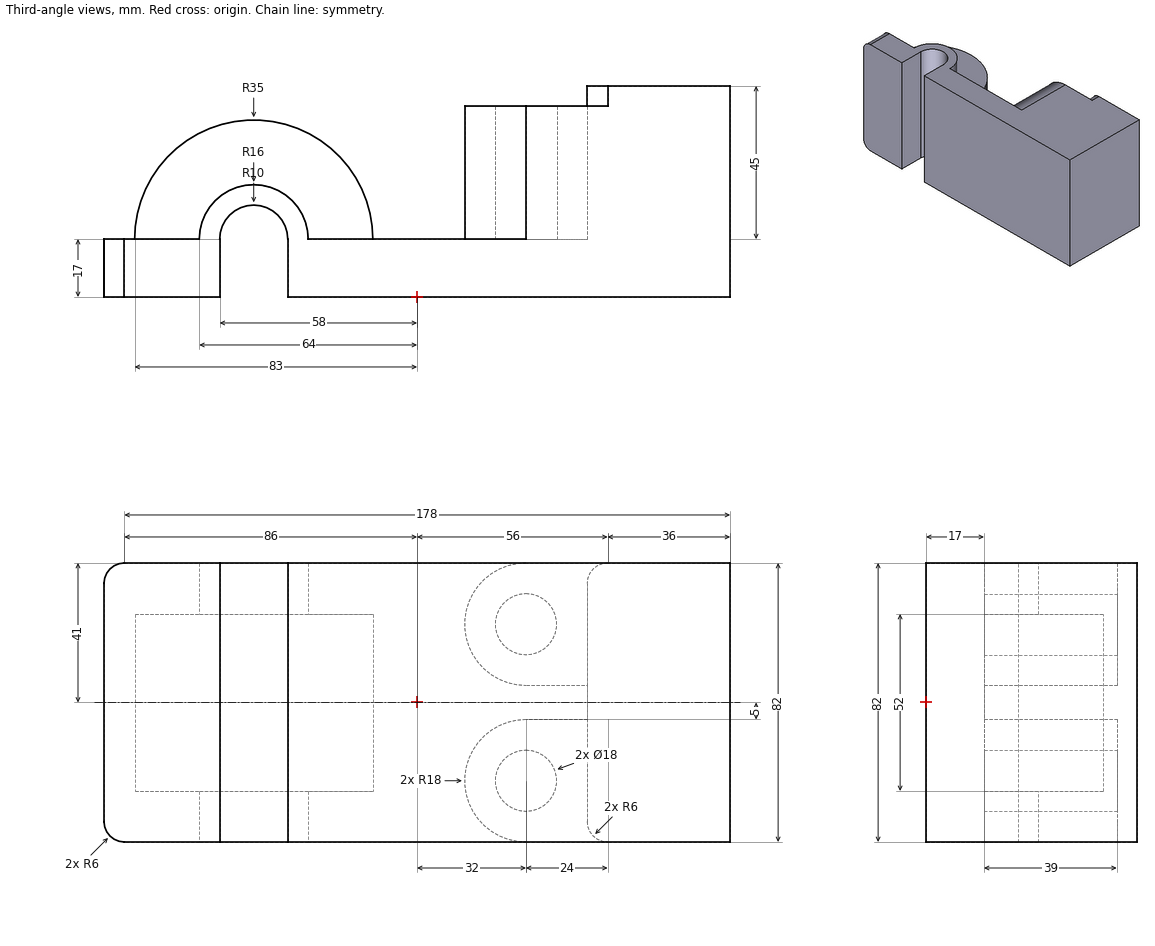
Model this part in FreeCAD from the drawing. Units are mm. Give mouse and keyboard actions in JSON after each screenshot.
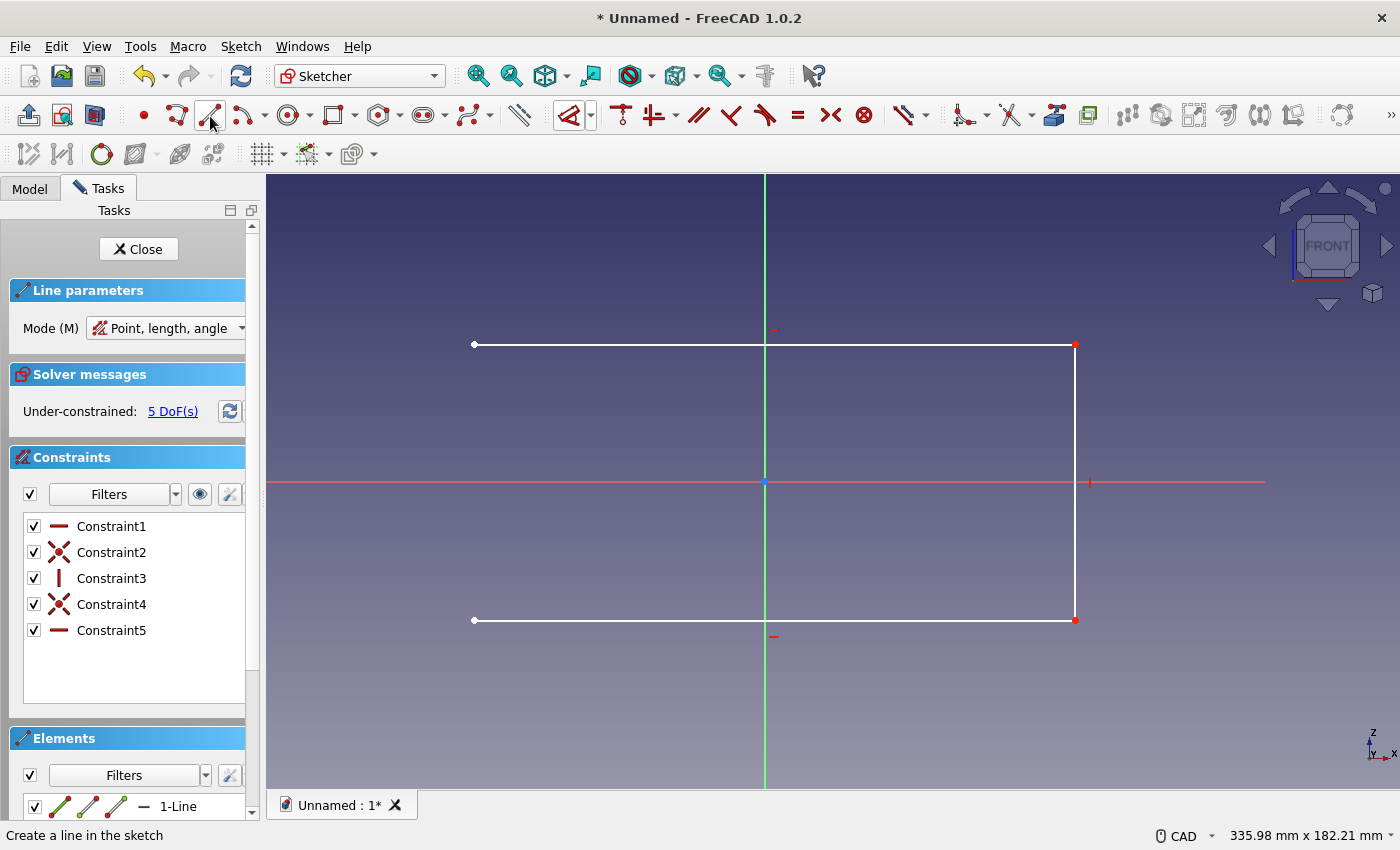
{"action": "left_click", "coordinate": [454, 600]}
{"action": "left_click", "coordinate": [454, 364]}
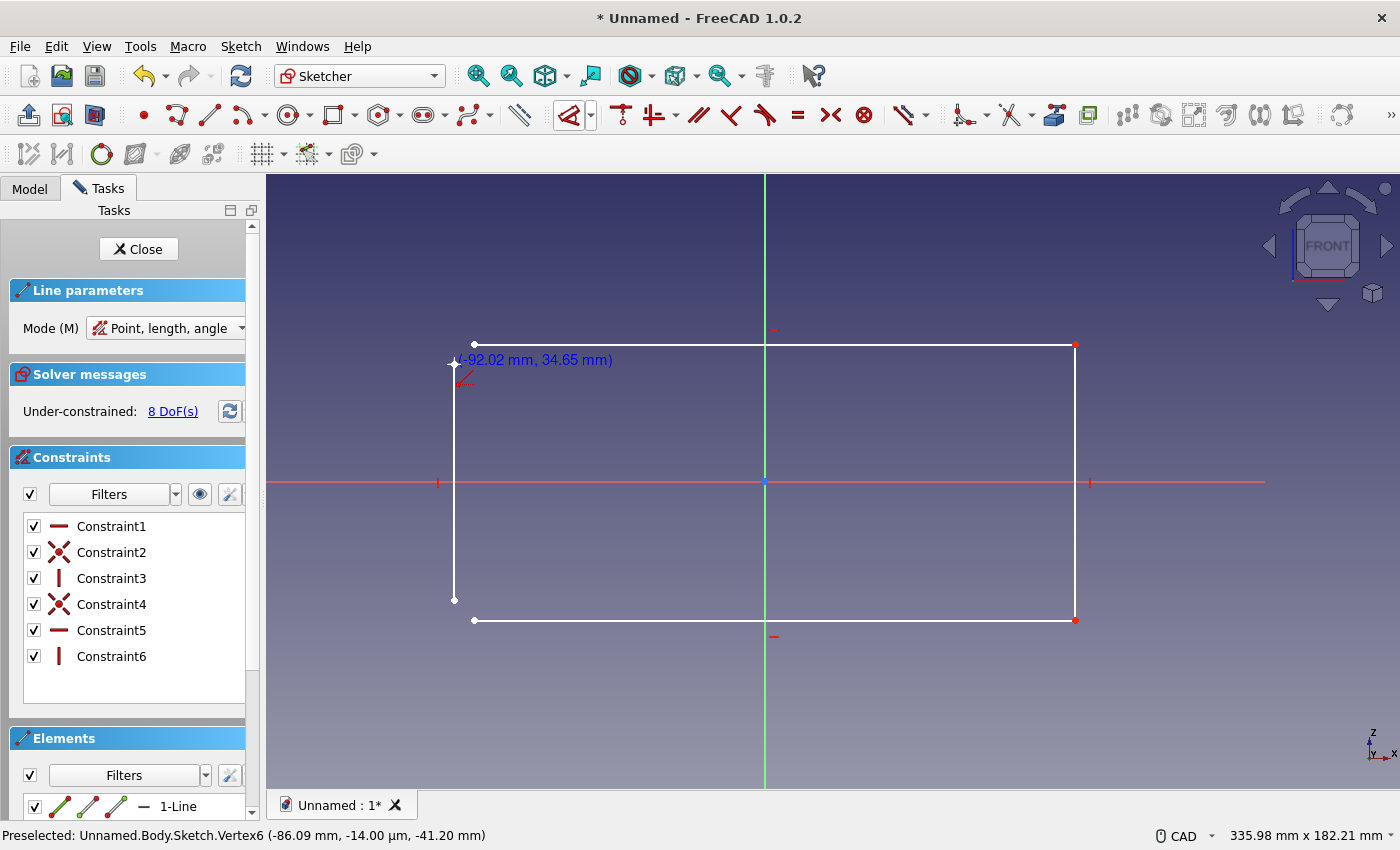
{"action": "key", "text": "g 3 a"}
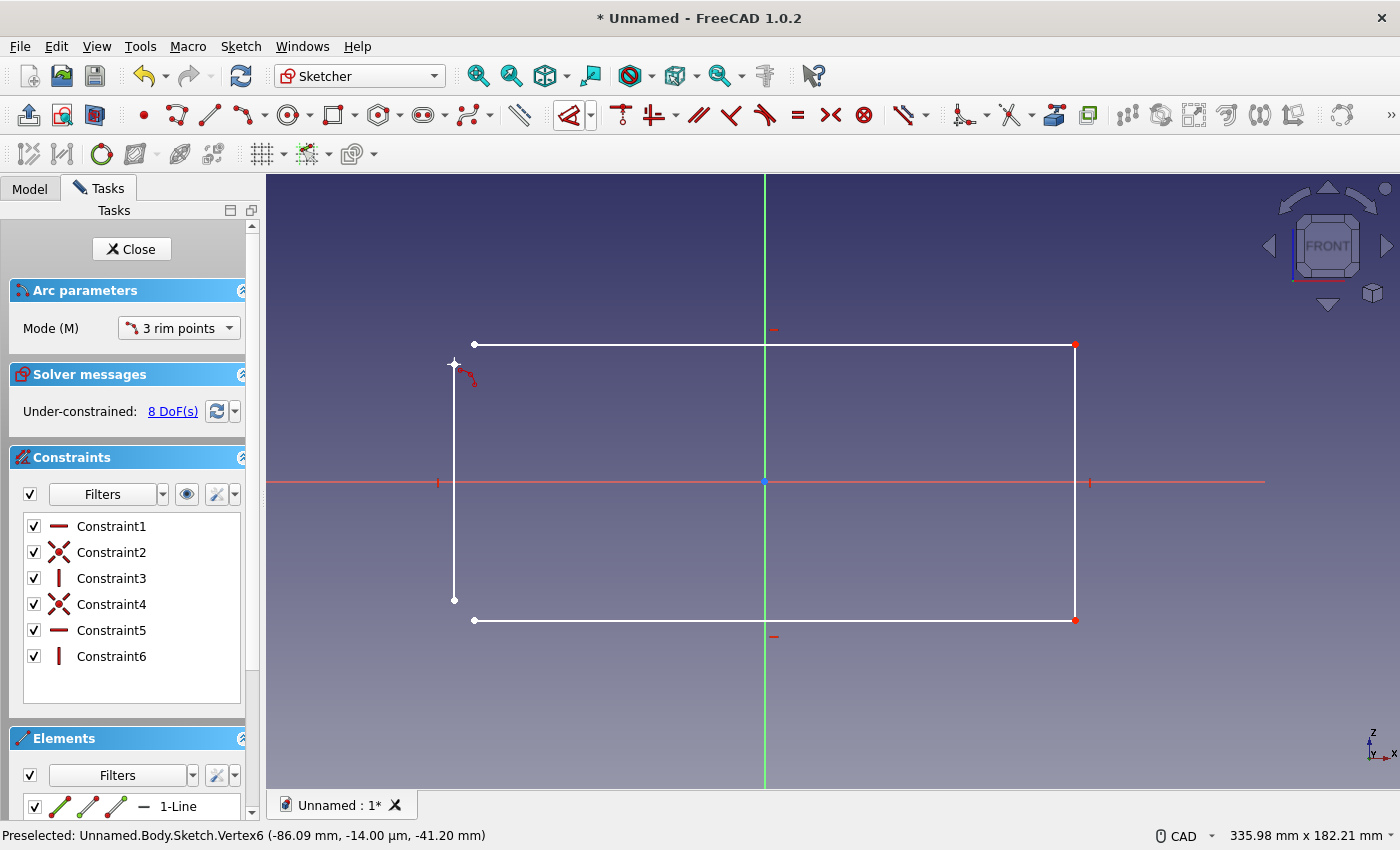
{"action": "left_click", "coordinate": [474, 621]}
{"action": "left_click", "coordinate": [454, 601]}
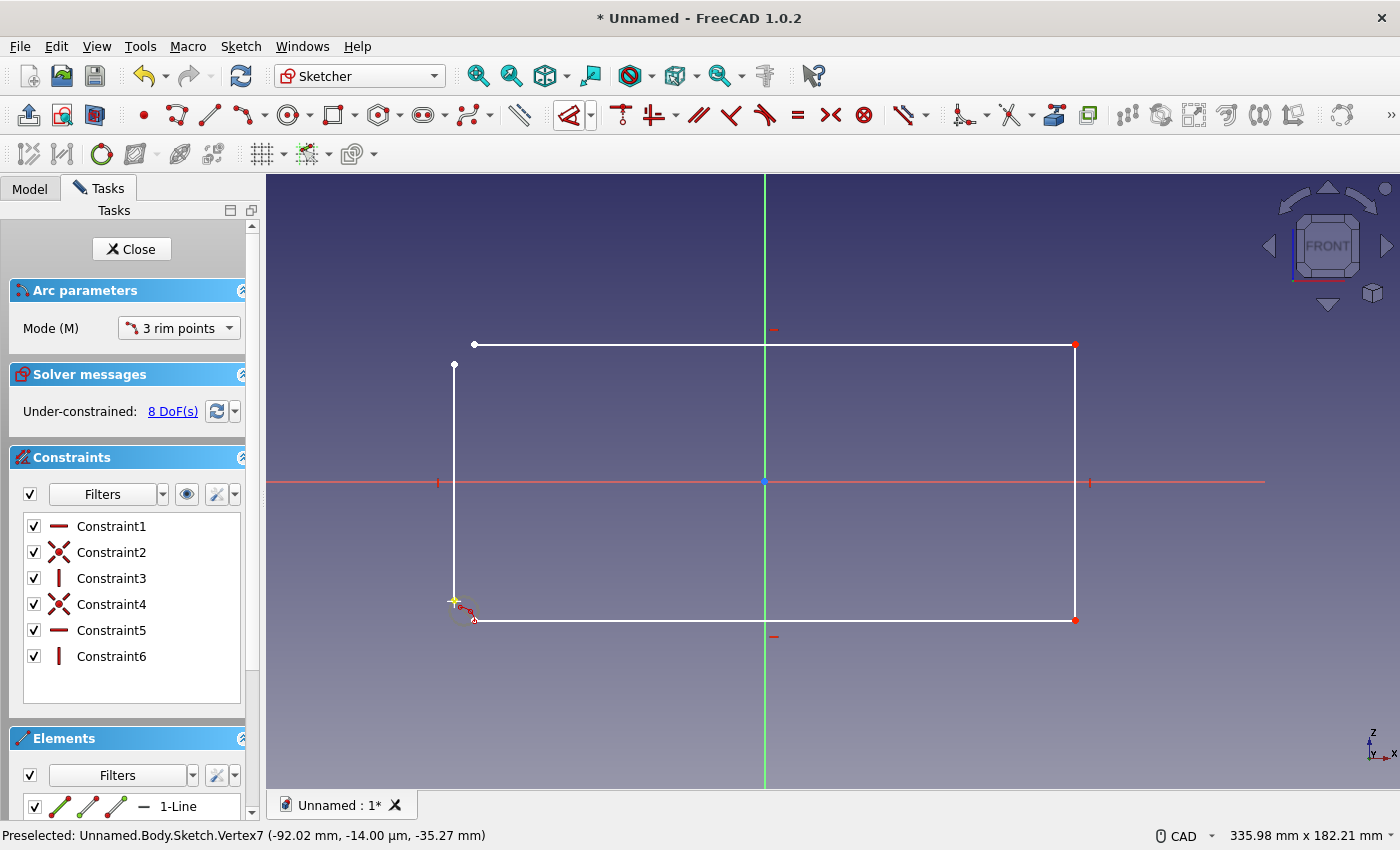
{"action": "scroll", "coordinate": [460, 614], "scroll_direction": "up", "scroll_amount": 5}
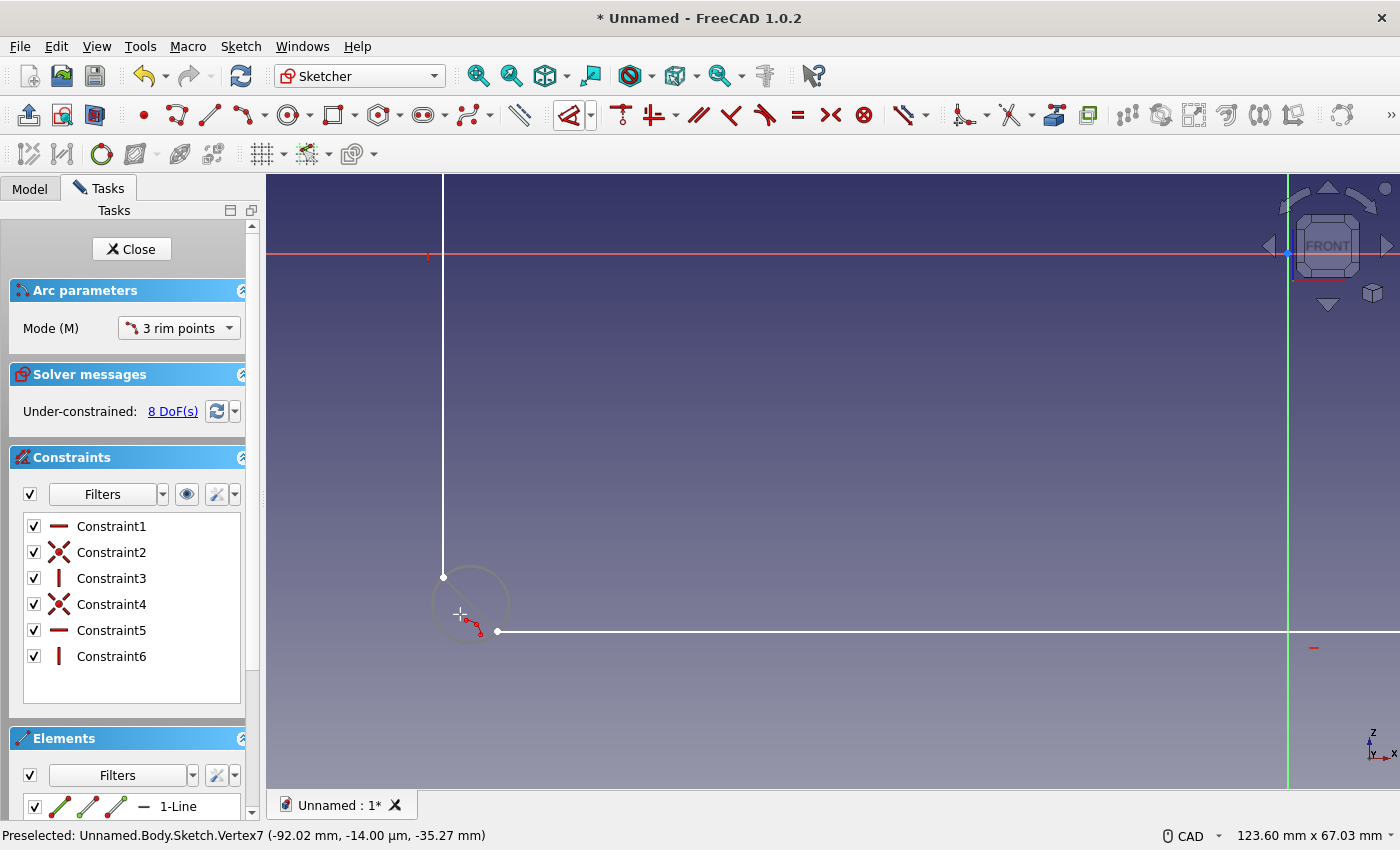
{"action": "left_click", "coordinate": [460, 614]}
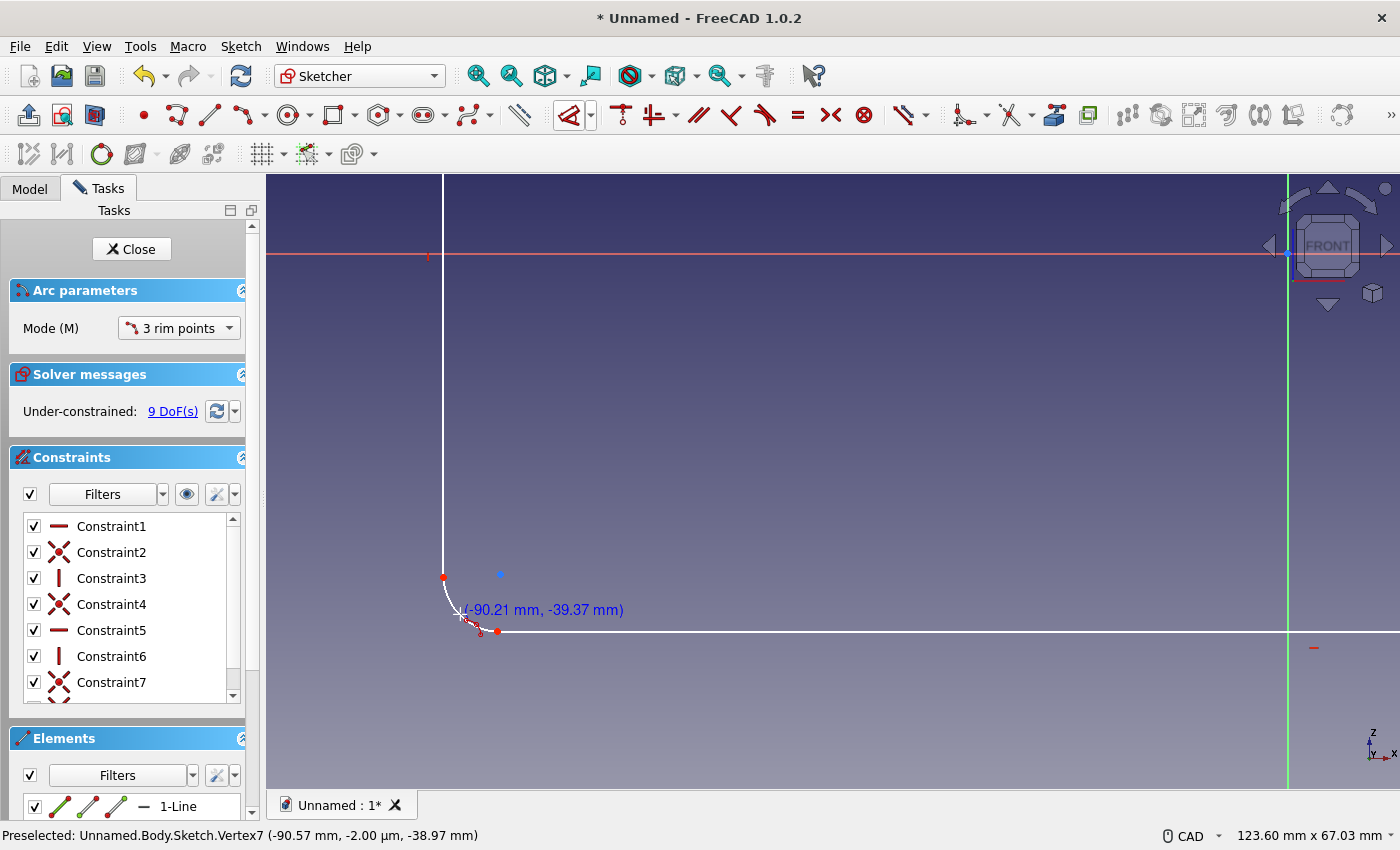
{"action": "scroll", "coordinate": [460, 614], "scroll_direction": "down", "scroll_amount": 5}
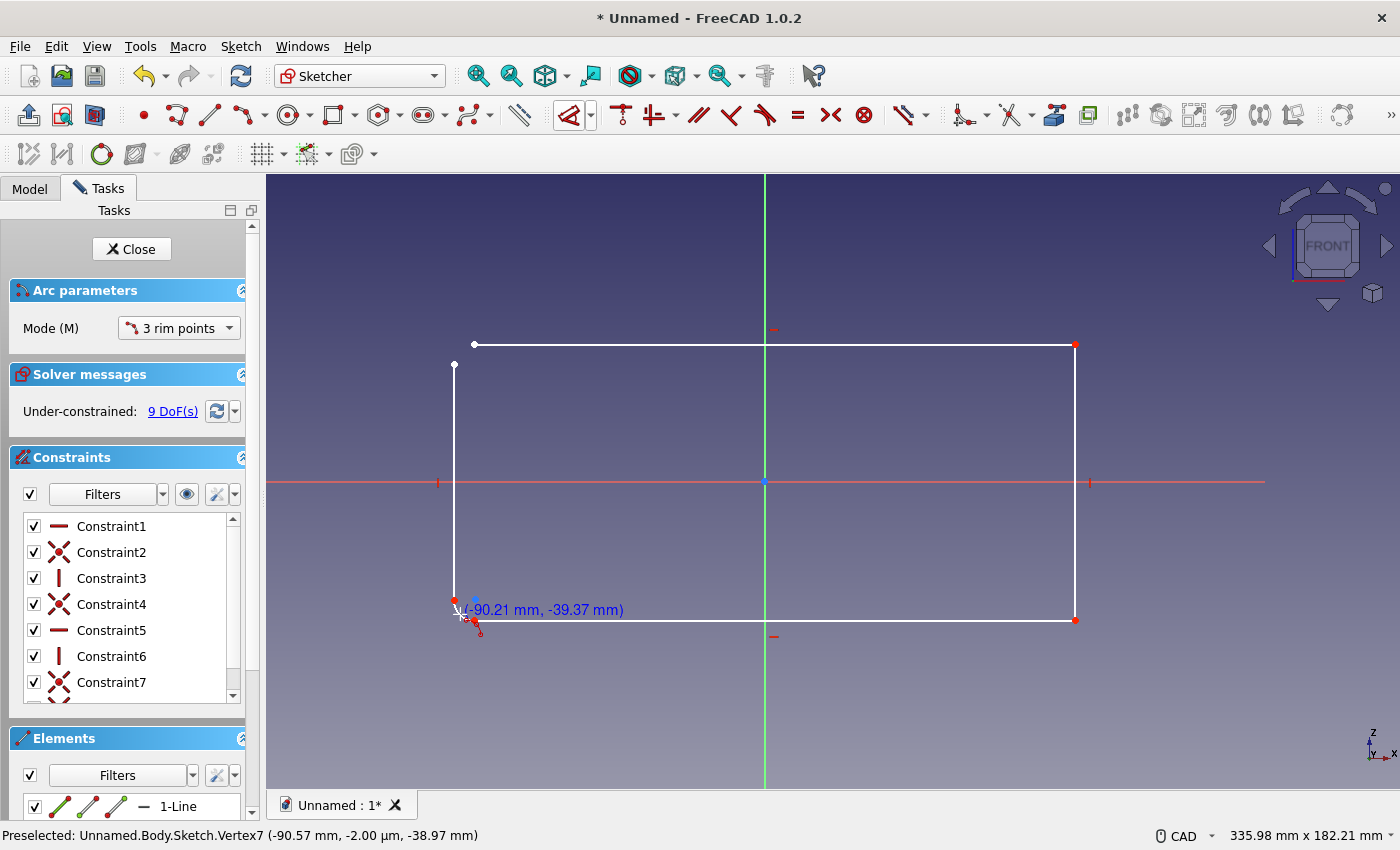
{"action": "left_click", "coordinate": [454, 365]}
{"action": "left_click", "coordinate": [474, 345]}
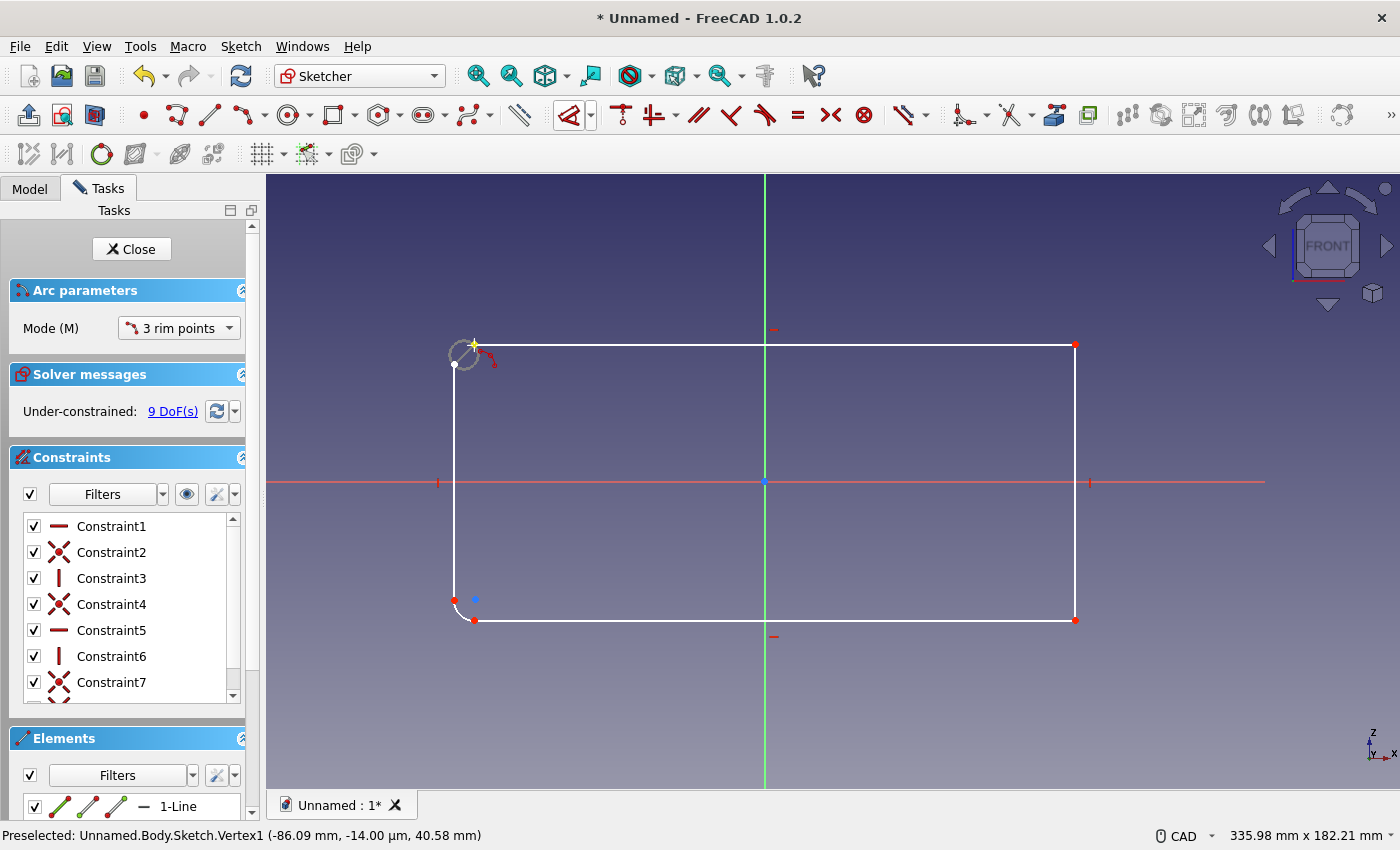
{"action": "scroll", "coordinate": [460, 350], "scroll_direction": "up", "scroll_amount": 5}